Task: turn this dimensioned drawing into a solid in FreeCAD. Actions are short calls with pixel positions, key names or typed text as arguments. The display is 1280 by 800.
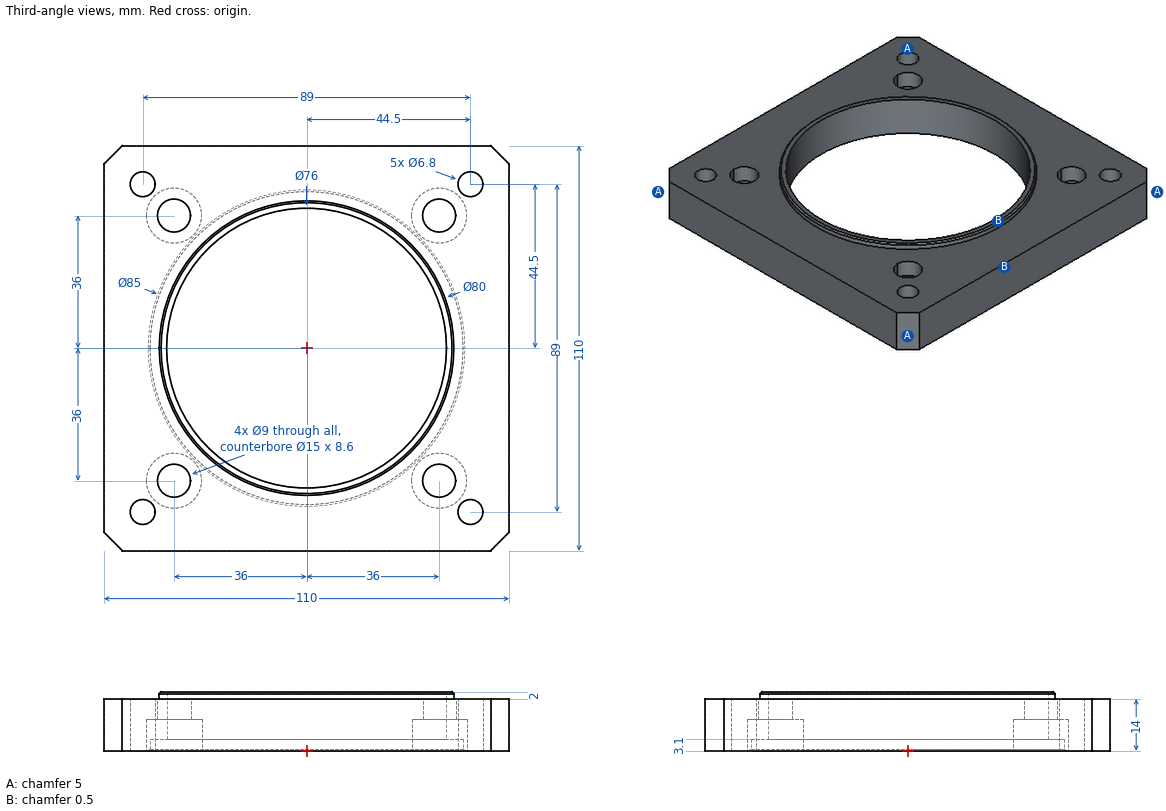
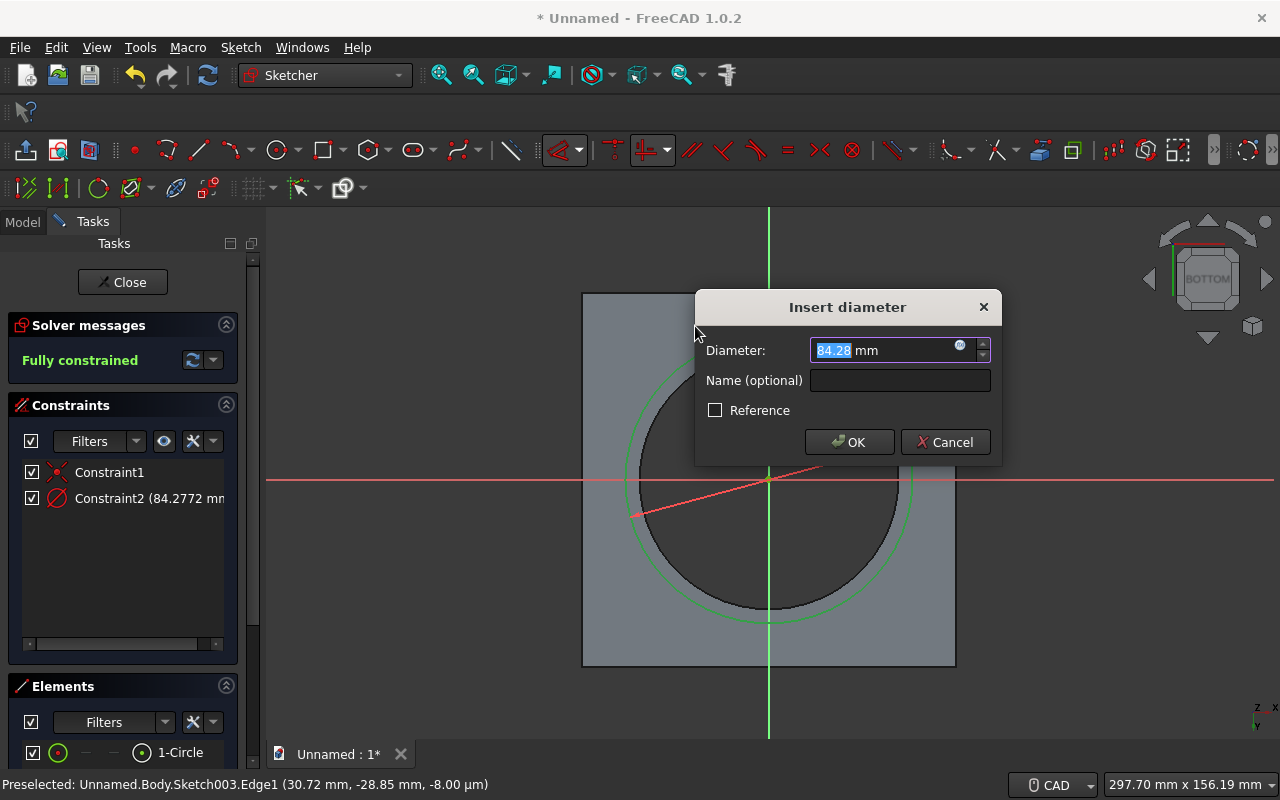
text(85)
key(Return)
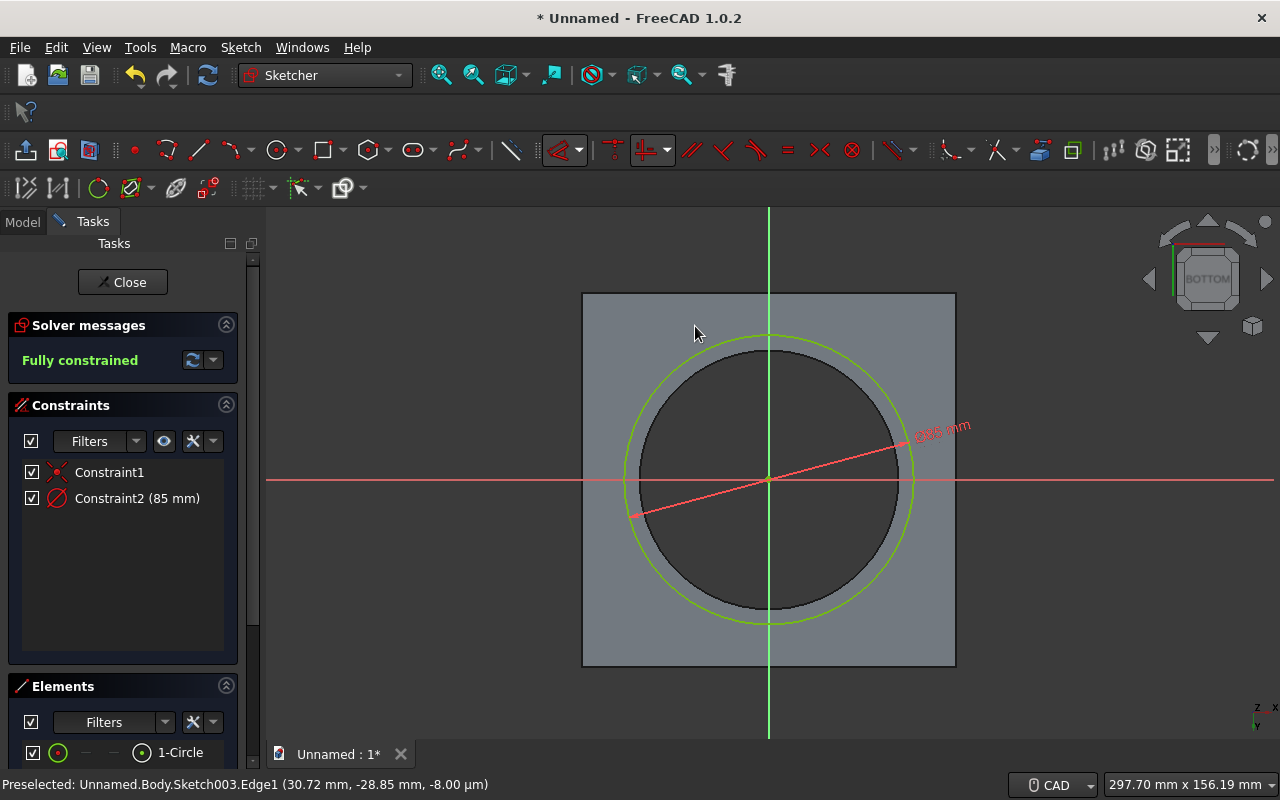
click(123, 282)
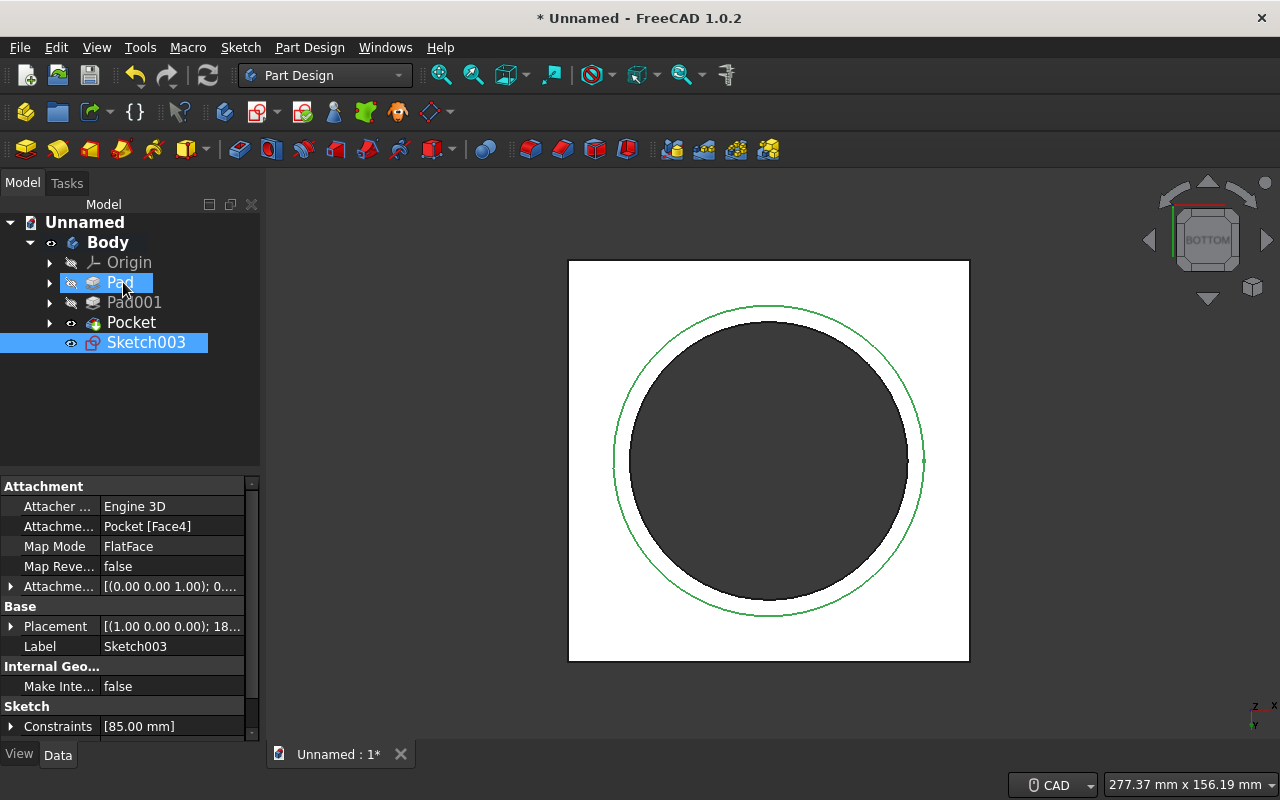
click(240, 150)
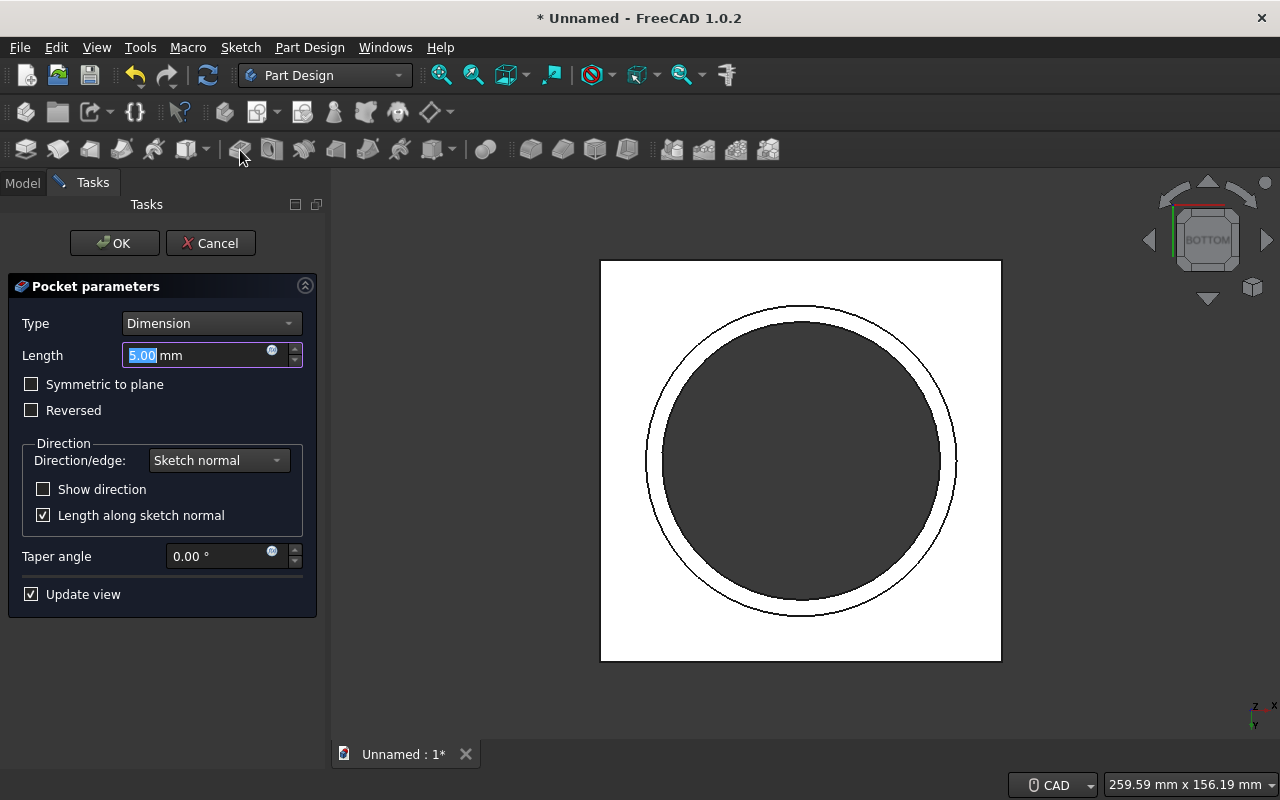
text(3.1)
key(Tab)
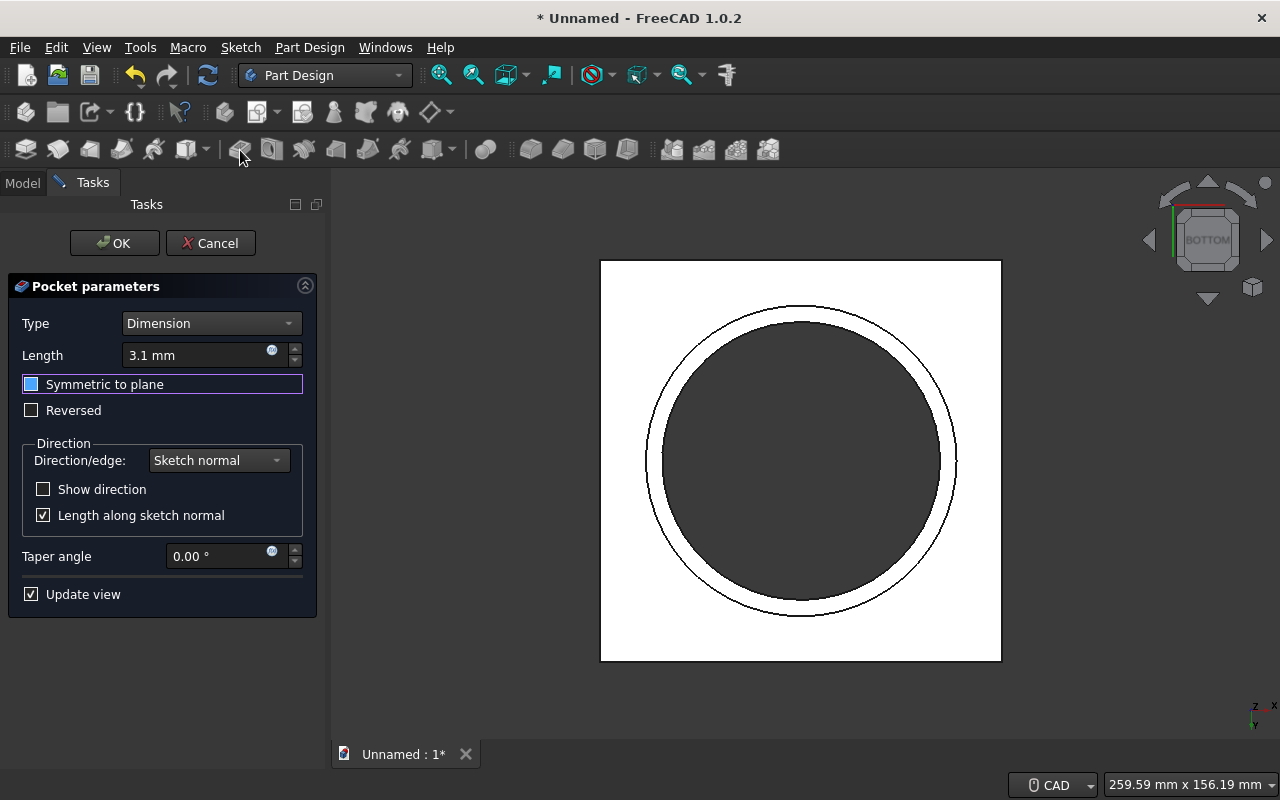
click(115, 243)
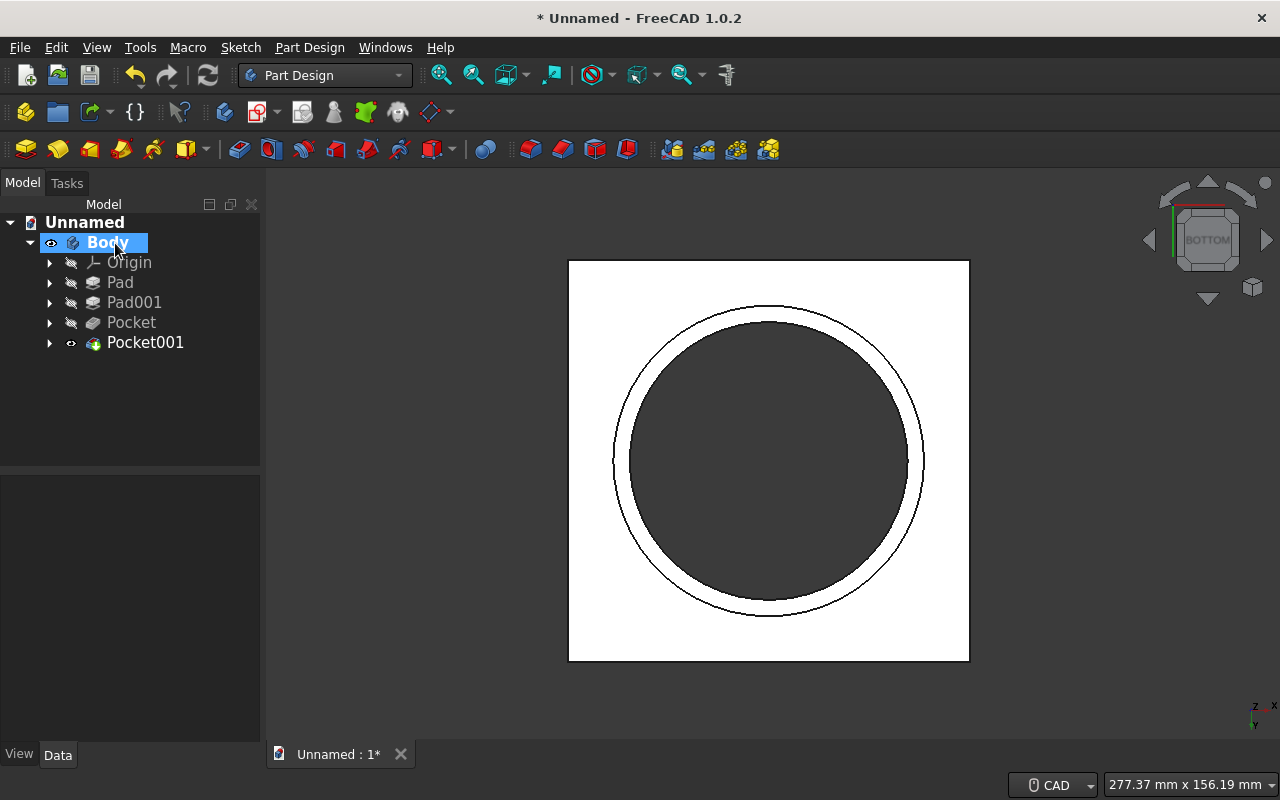
click(941, 632)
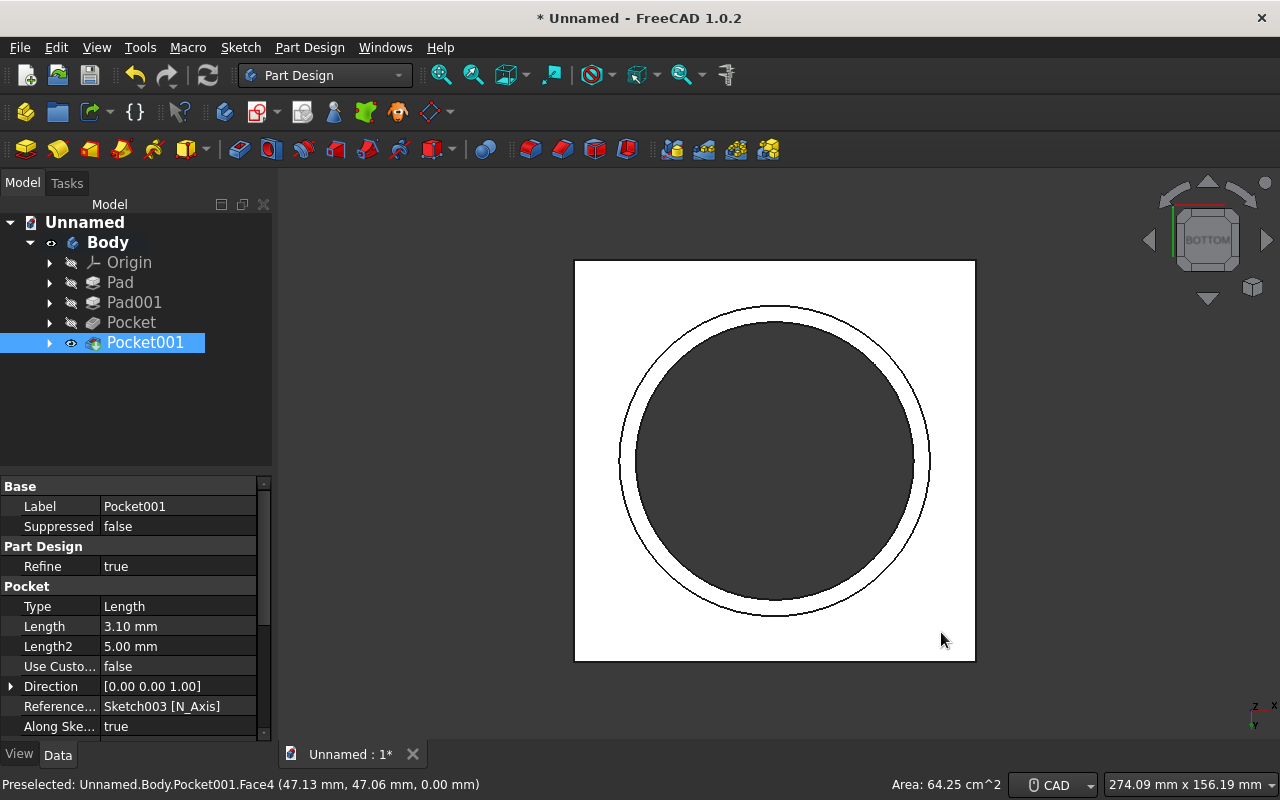
click(258, 112)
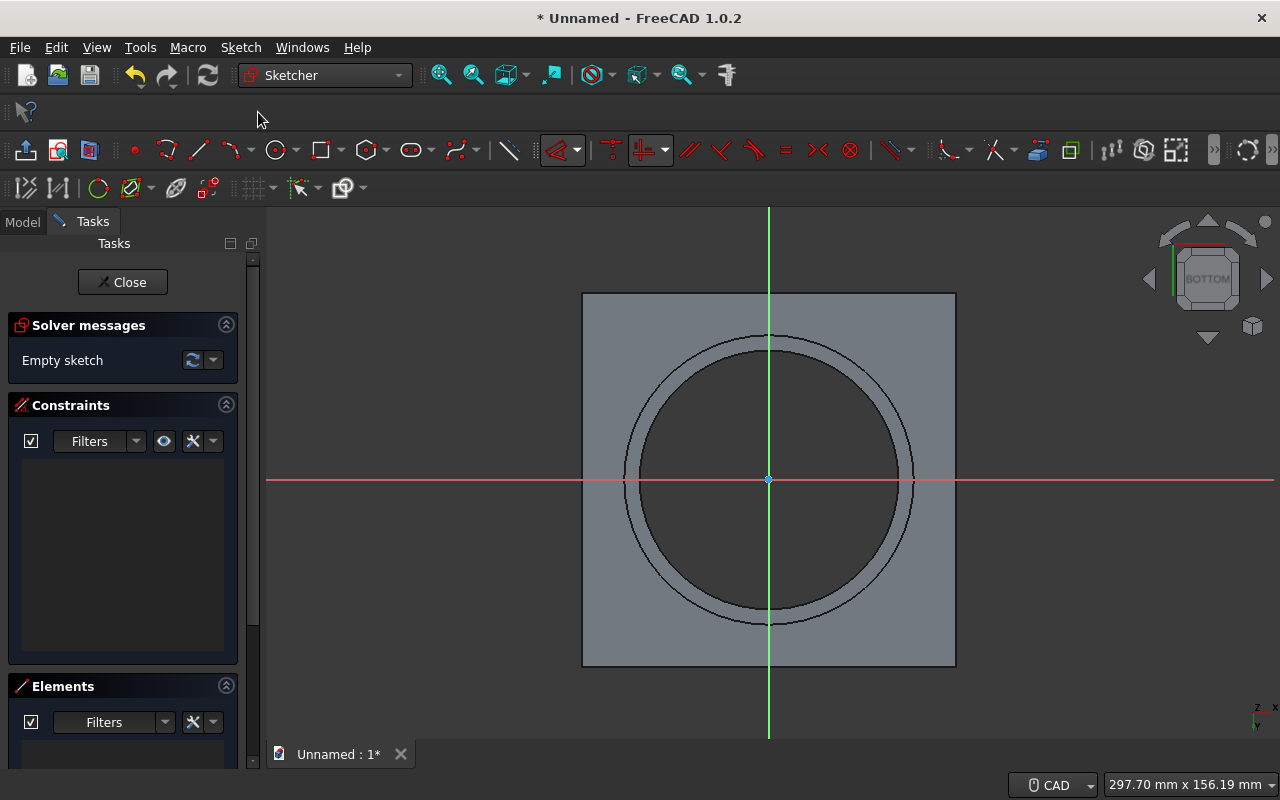
click(276, 150)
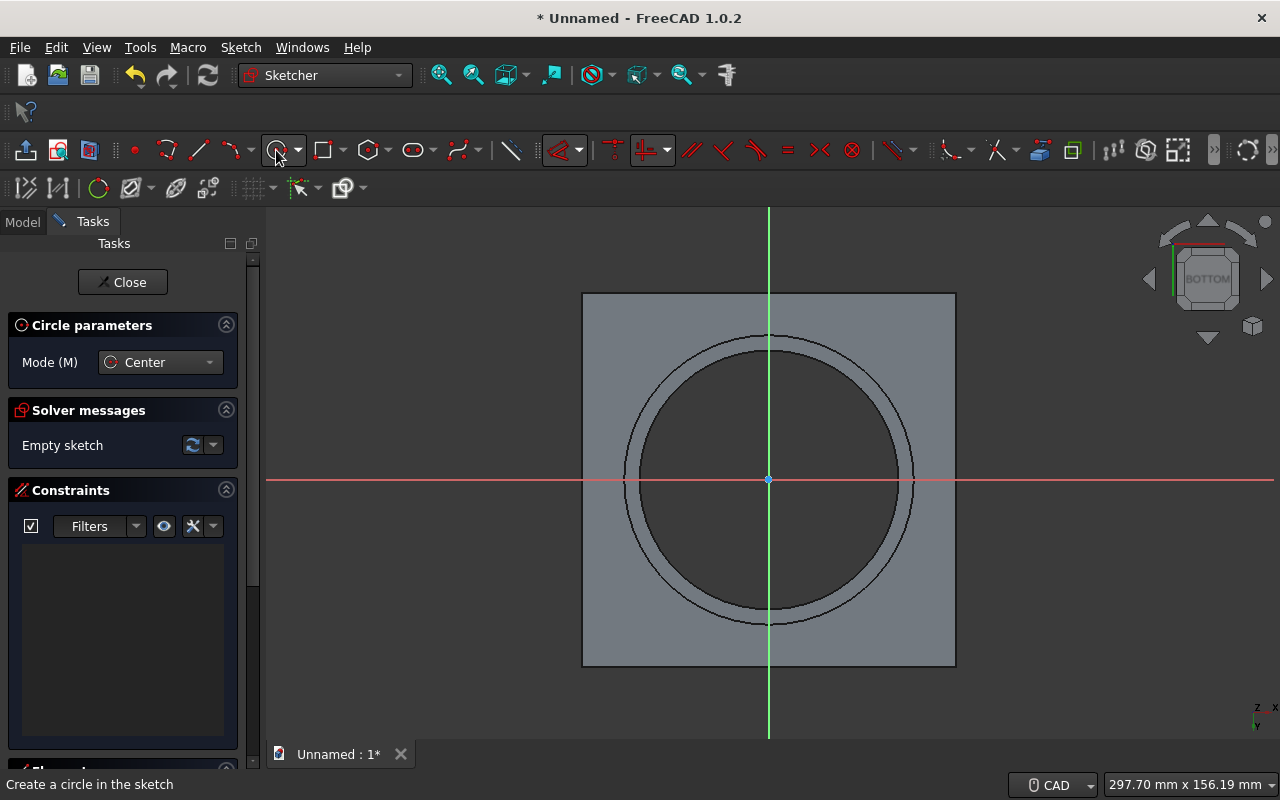
scroll(921, 632, up, 4)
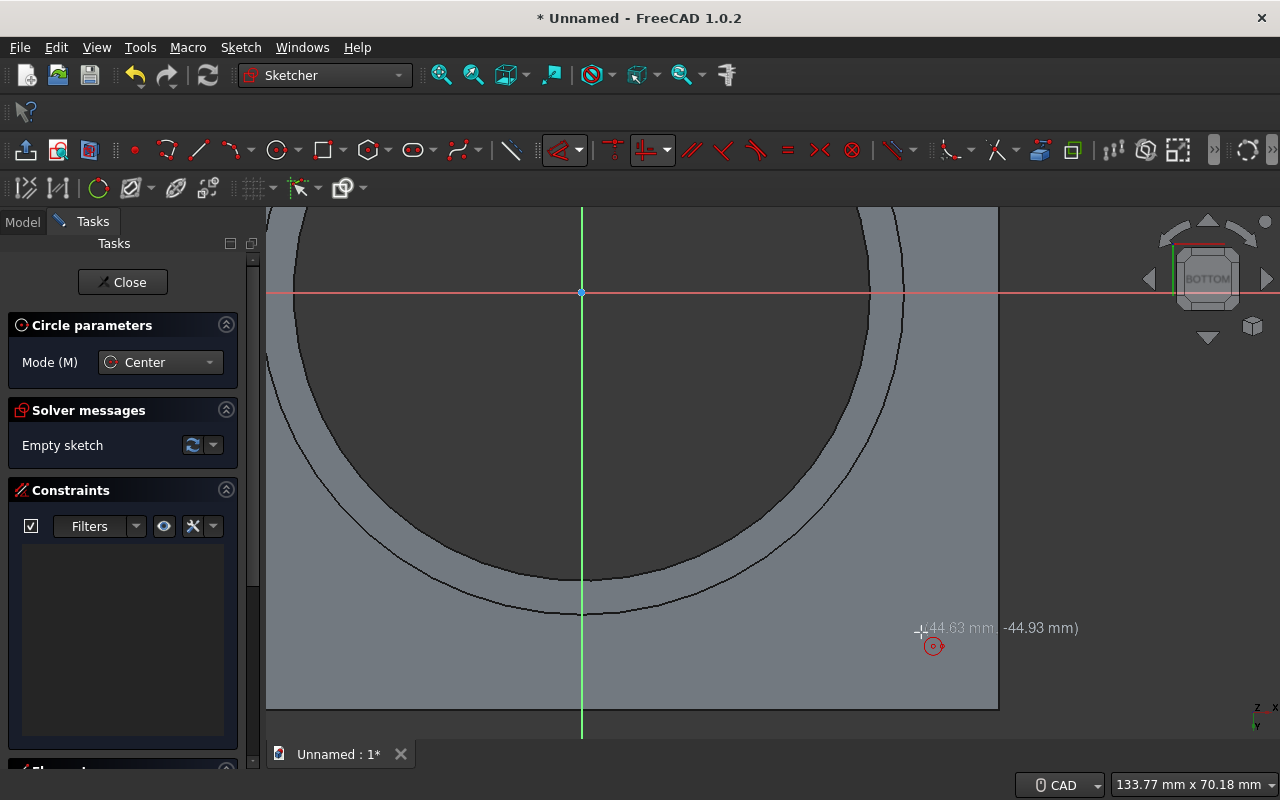
click(919, 630)
click(937, 612)